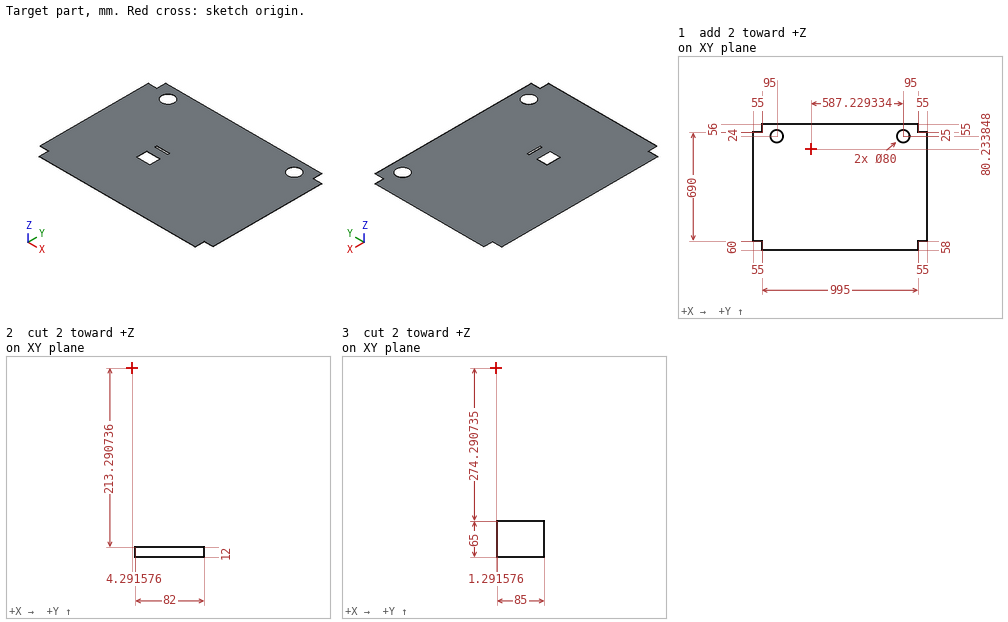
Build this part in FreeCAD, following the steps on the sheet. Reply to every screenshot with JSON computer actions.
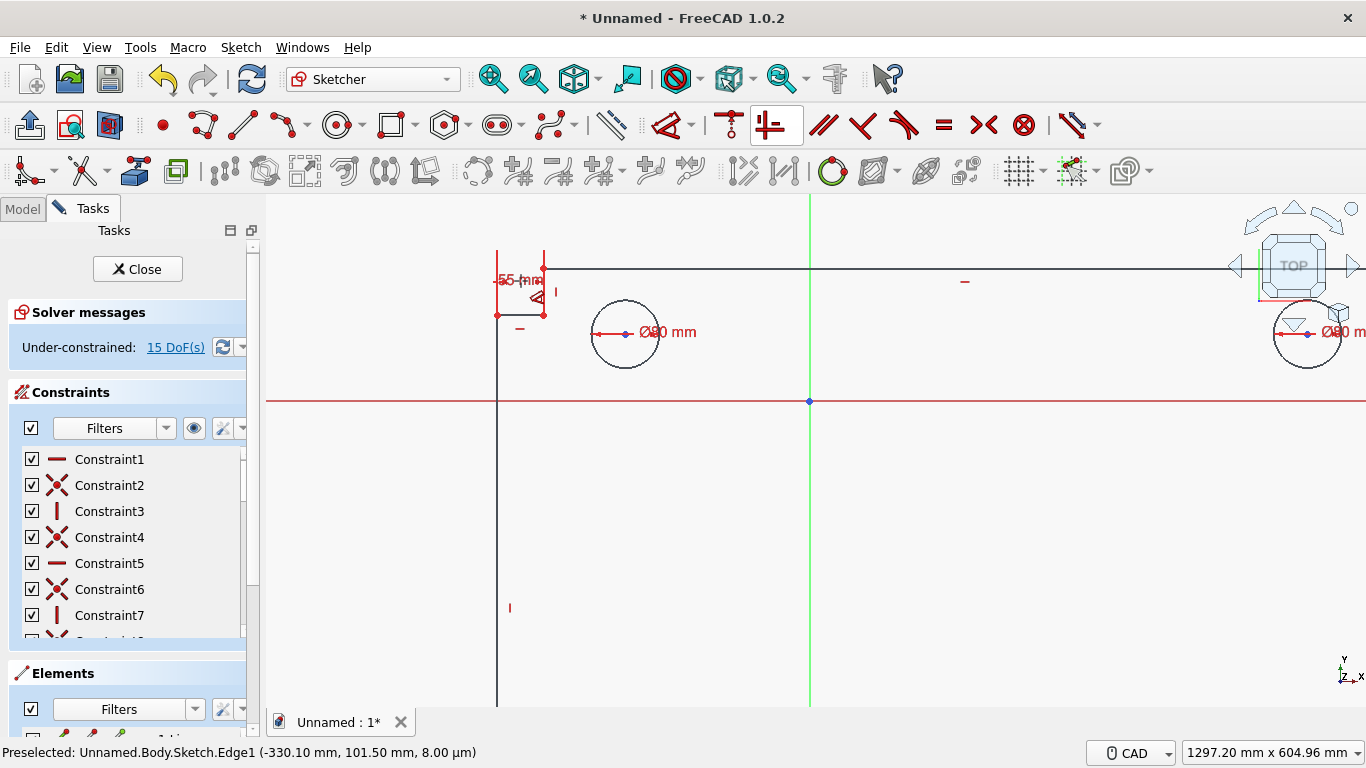
{"action": "scroll", "coordinate": [569, 323], "scroll_direction": "down", "scroll_amount": 4}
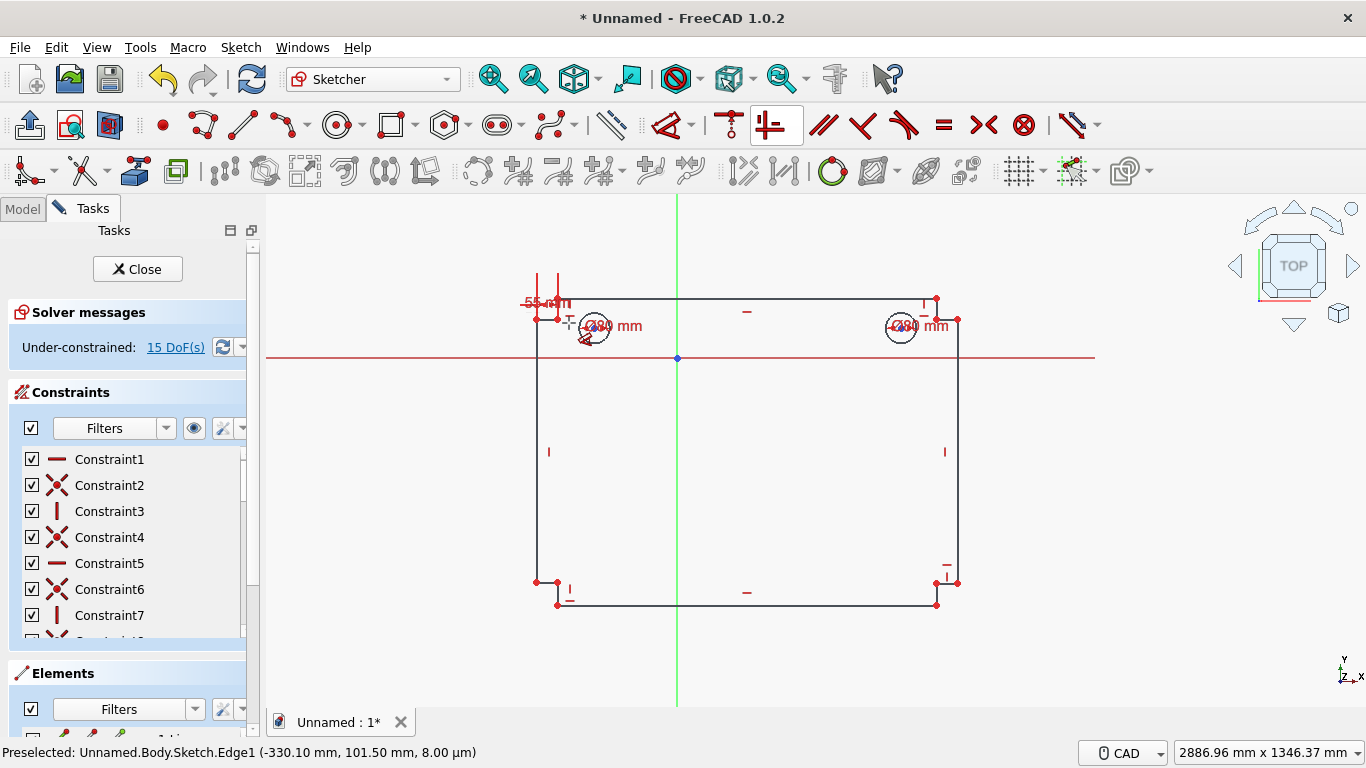
{"action": "scroll", "coordinate": [543, 583], "scroll_direction": "up", "scroll_amount": 4}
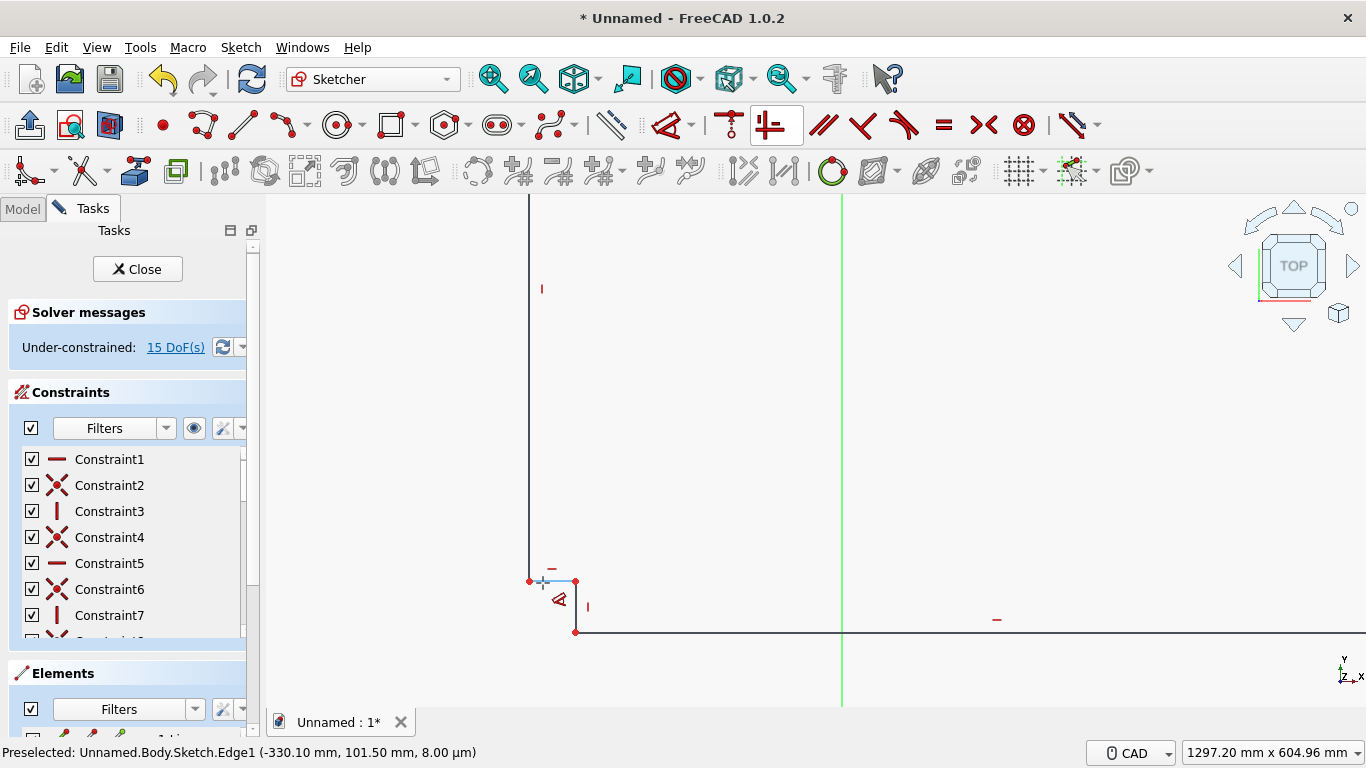
{"action": "left_click", "coordinate": [543, 581]}
{"action": "left_click", "coordinate": [553, 615]}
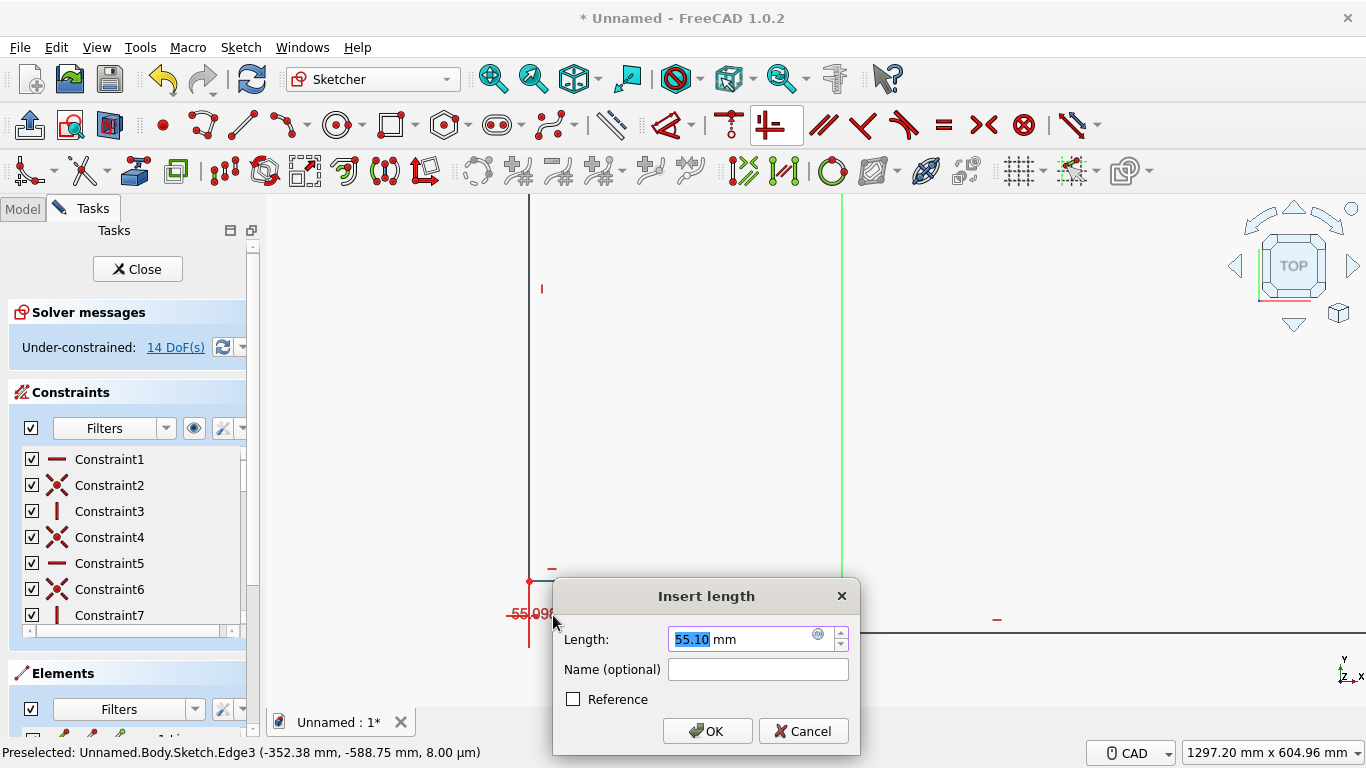
{"action": "type", "text": "55"}
{"action": "key", "text": "Return"}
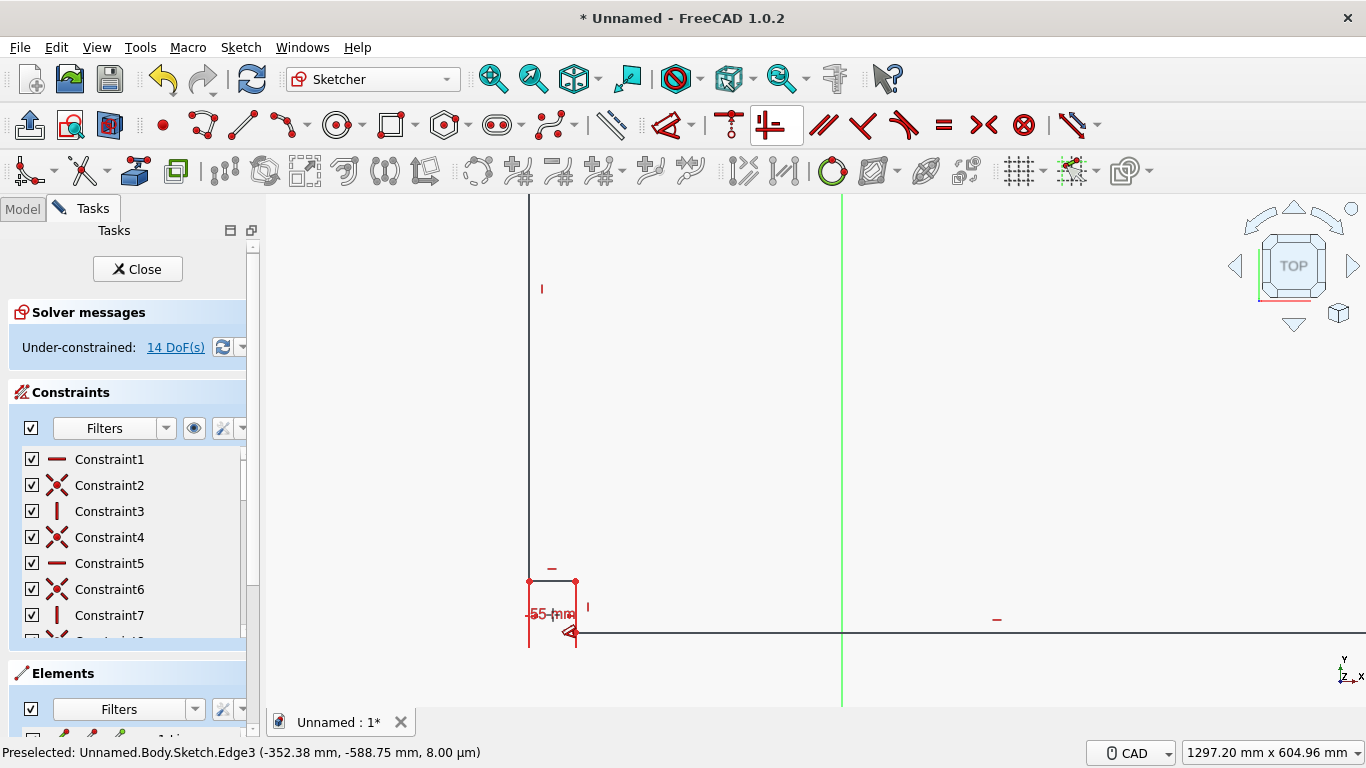
{"action": "left_click", "coordinate": [576, 597]}
{"action": "left_click", "coordinate": [542, 595]}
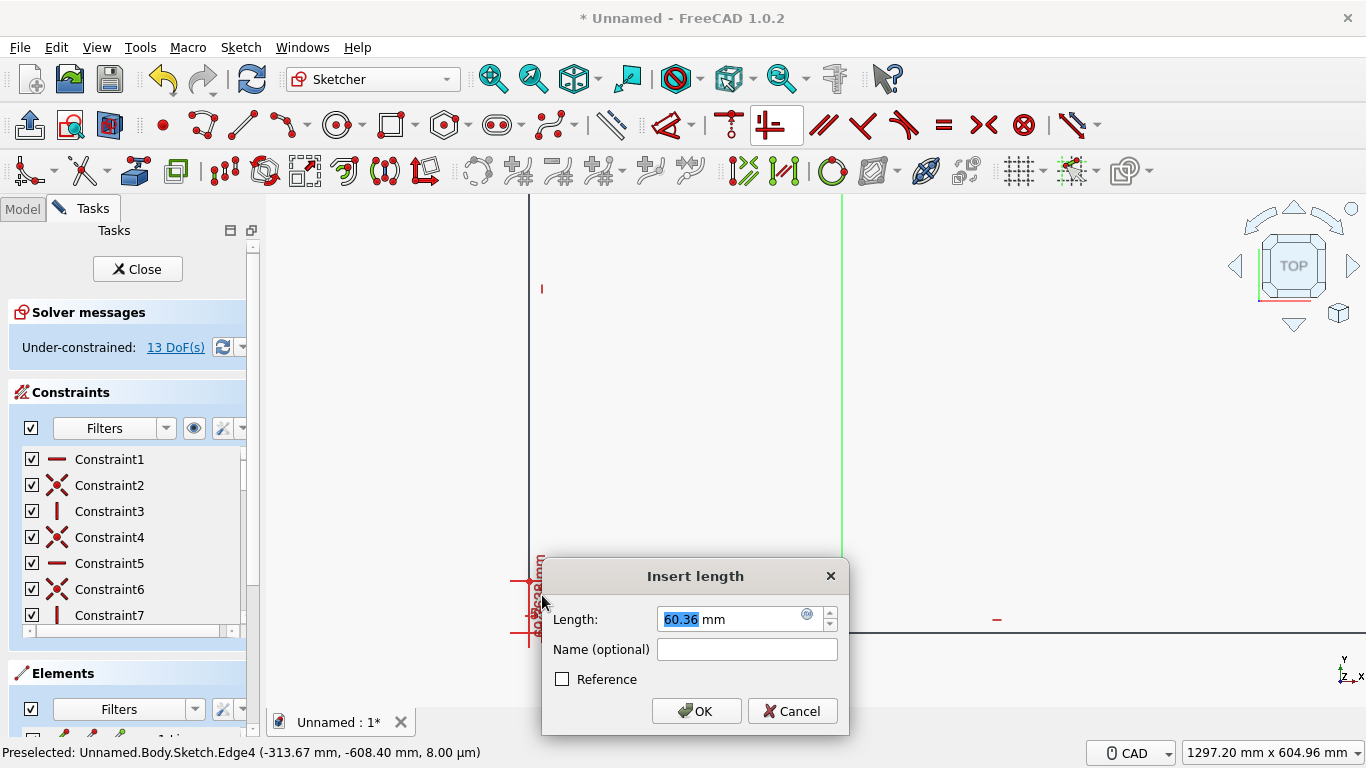
{"action": "type", "text": "60"}
{"action": "key", "text": "Return"}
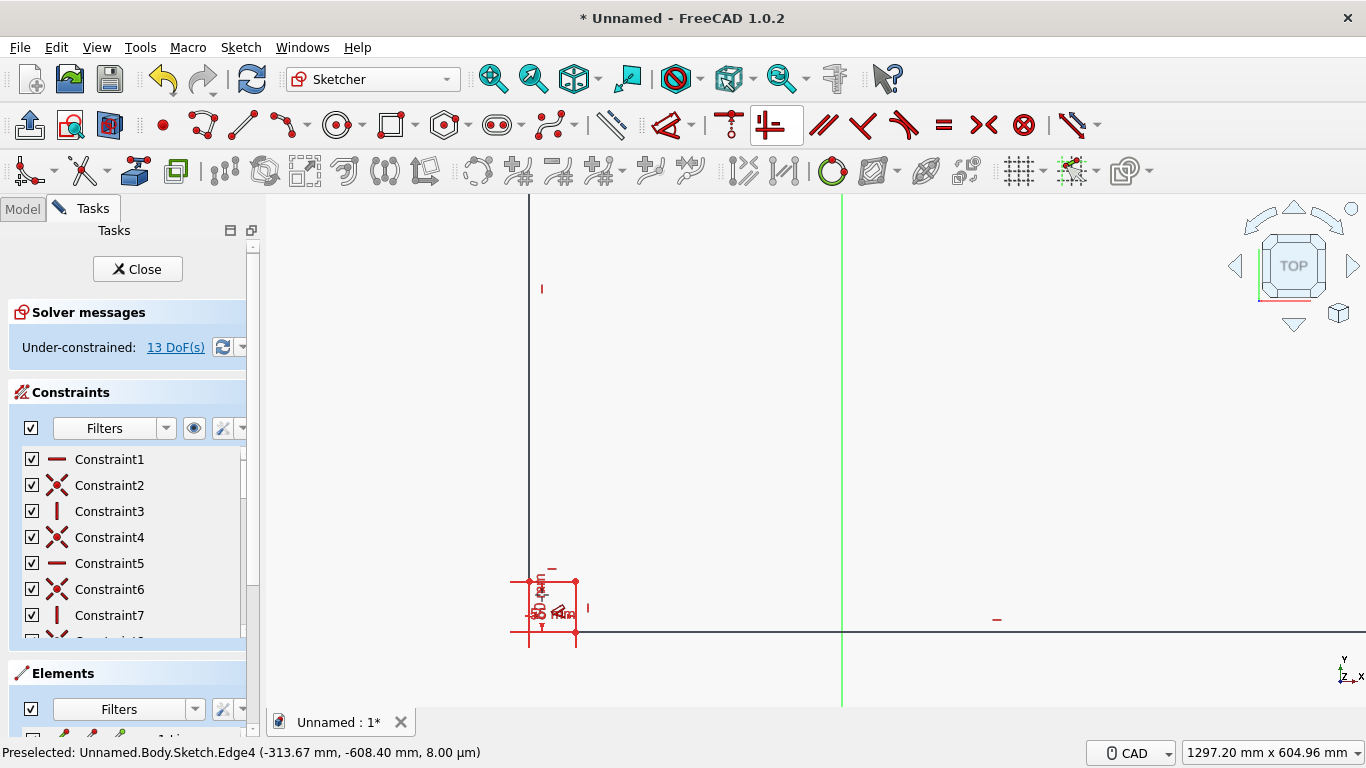
{"action": "scroll", "coordinate": [543, 583], "scroll_direction": "down", "scroll_amount": 4}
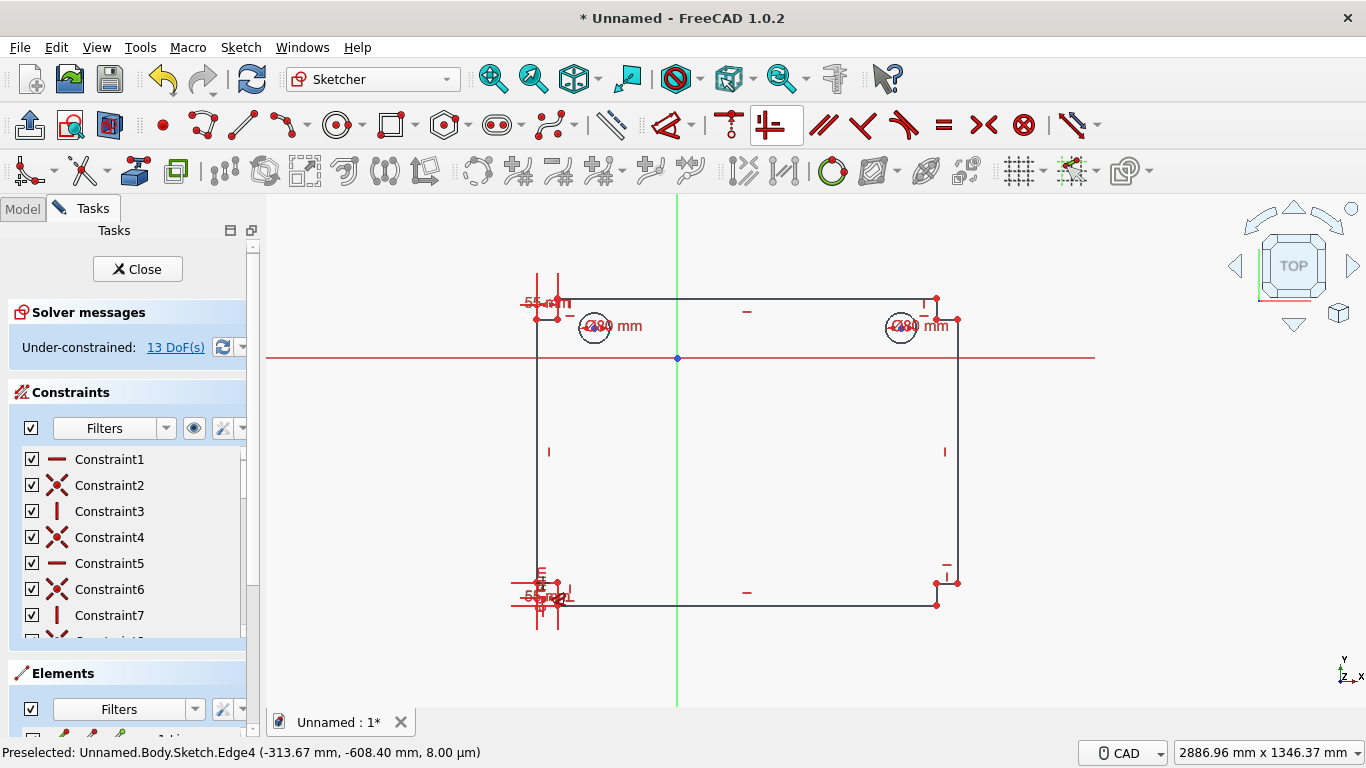
{"action": "scroll", "coordinate": [937, 599], "scroll_direction": "up", "scroll_amount": 4}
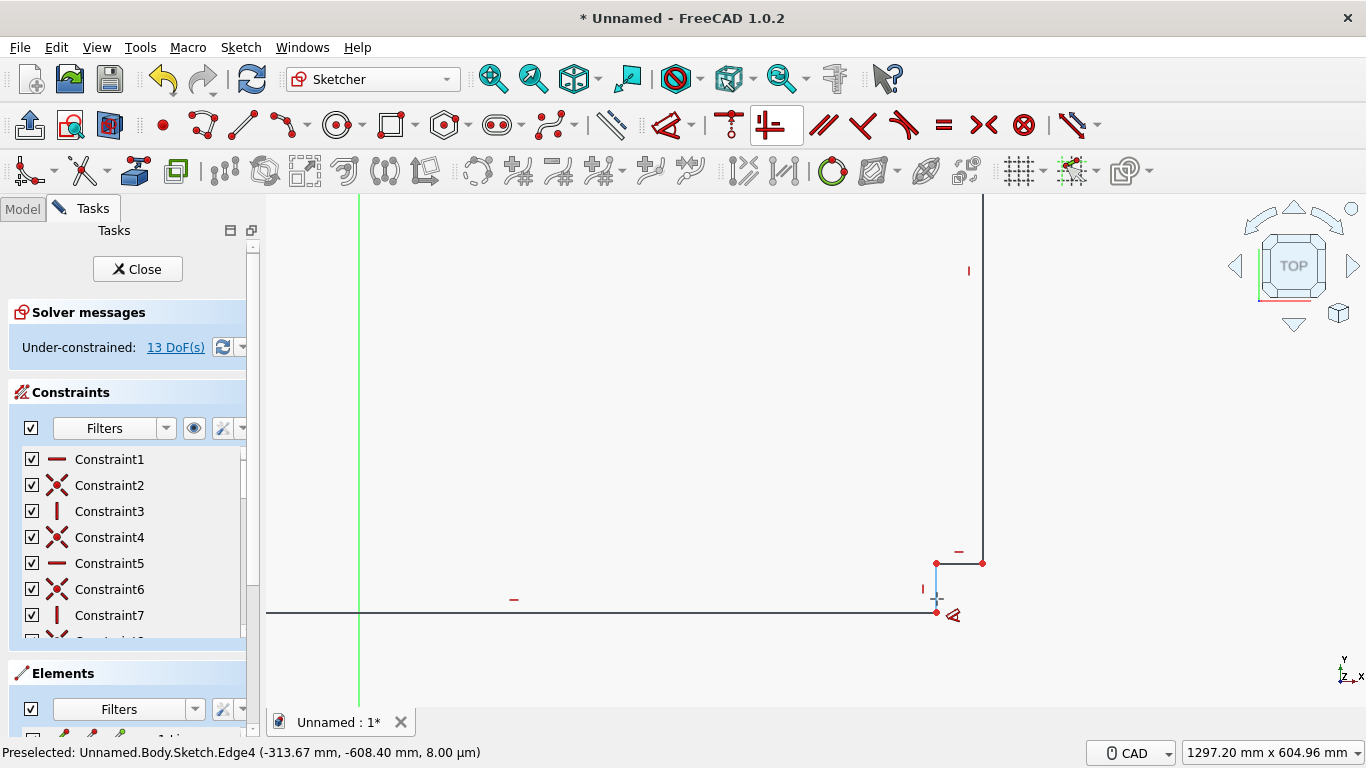
{"action": "left_click", "coordinate": [936, 598]}
{"action": "left_click", "coordinate": [970, 588]}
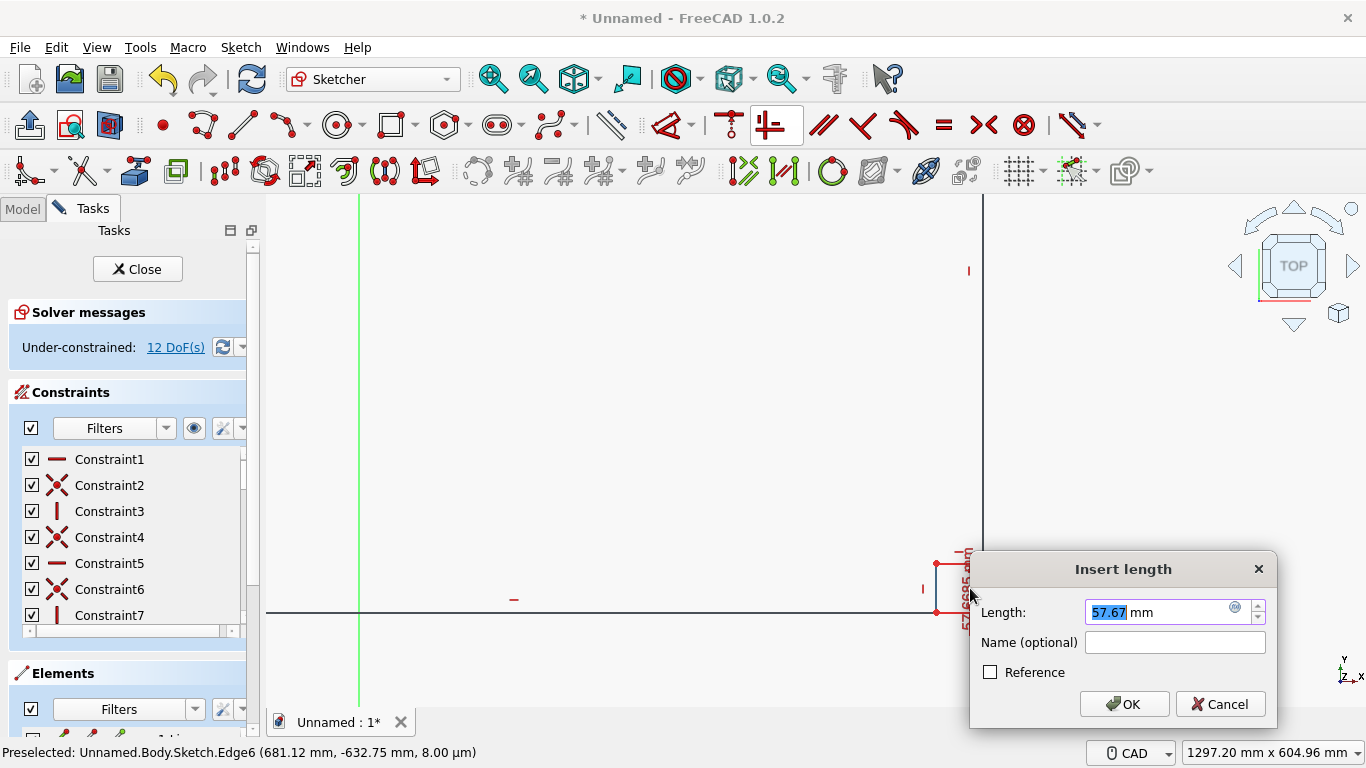
{"action": "type", "text": "58"}
{"action": "key", "text": "Return"}